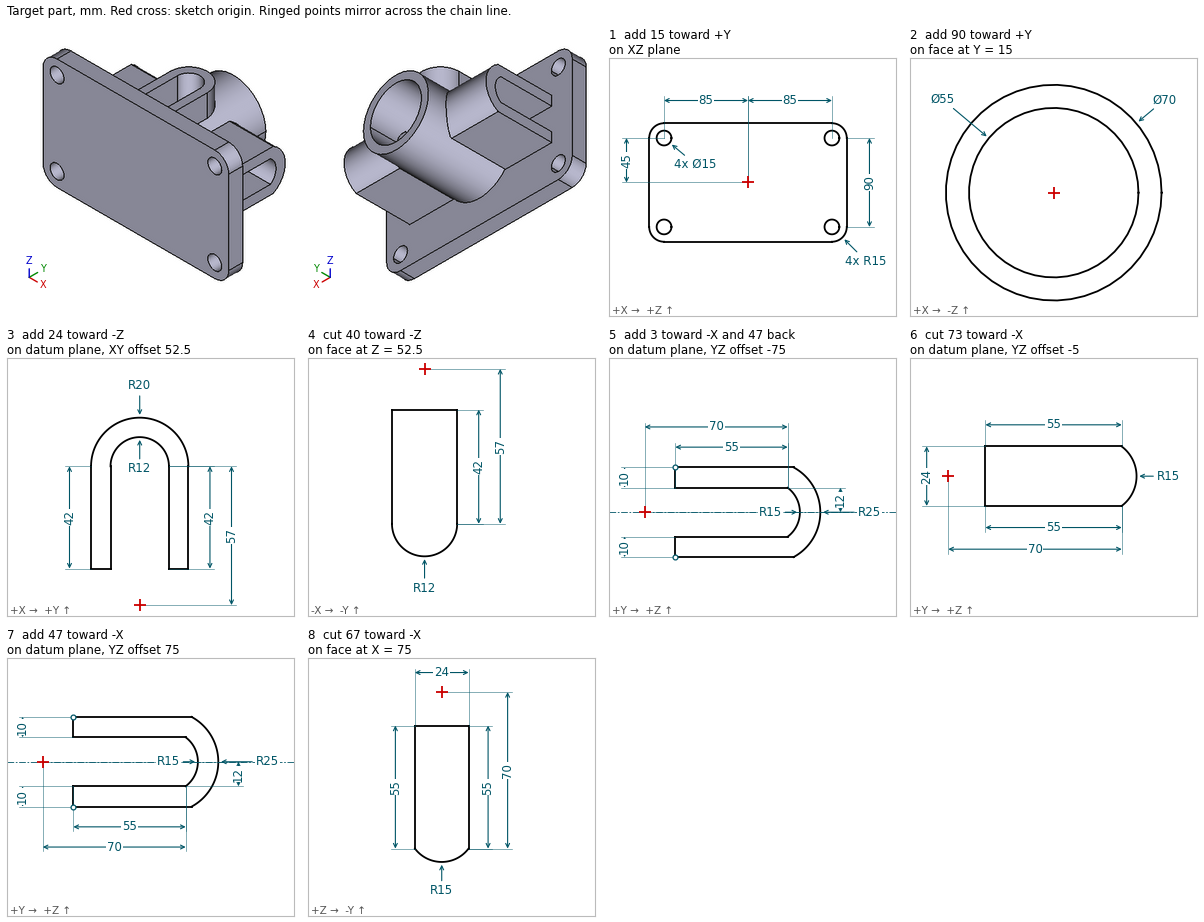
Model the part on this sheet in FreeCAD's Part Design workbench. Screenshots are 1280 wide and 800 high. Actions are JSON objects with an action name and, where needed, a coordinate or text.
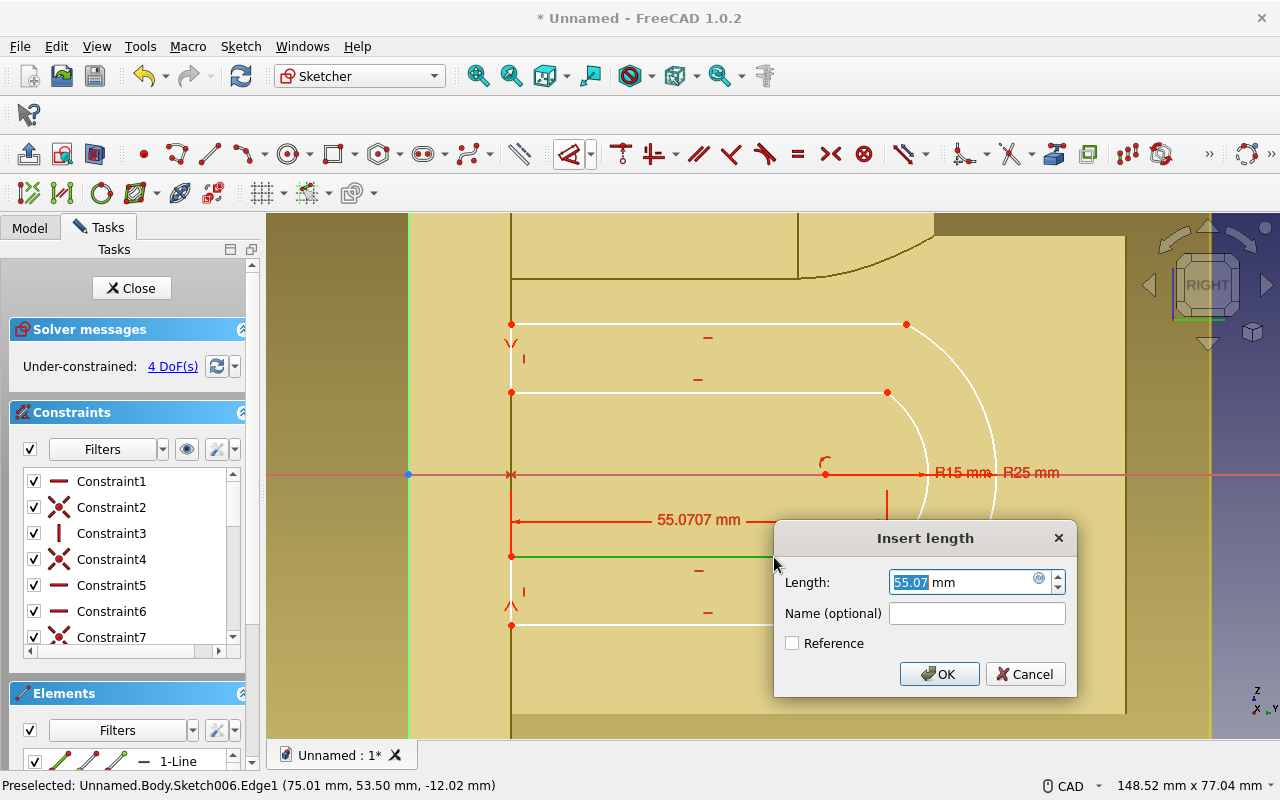
{"action": "type", "text": "55"}
{"action": "key", "text": "Return"}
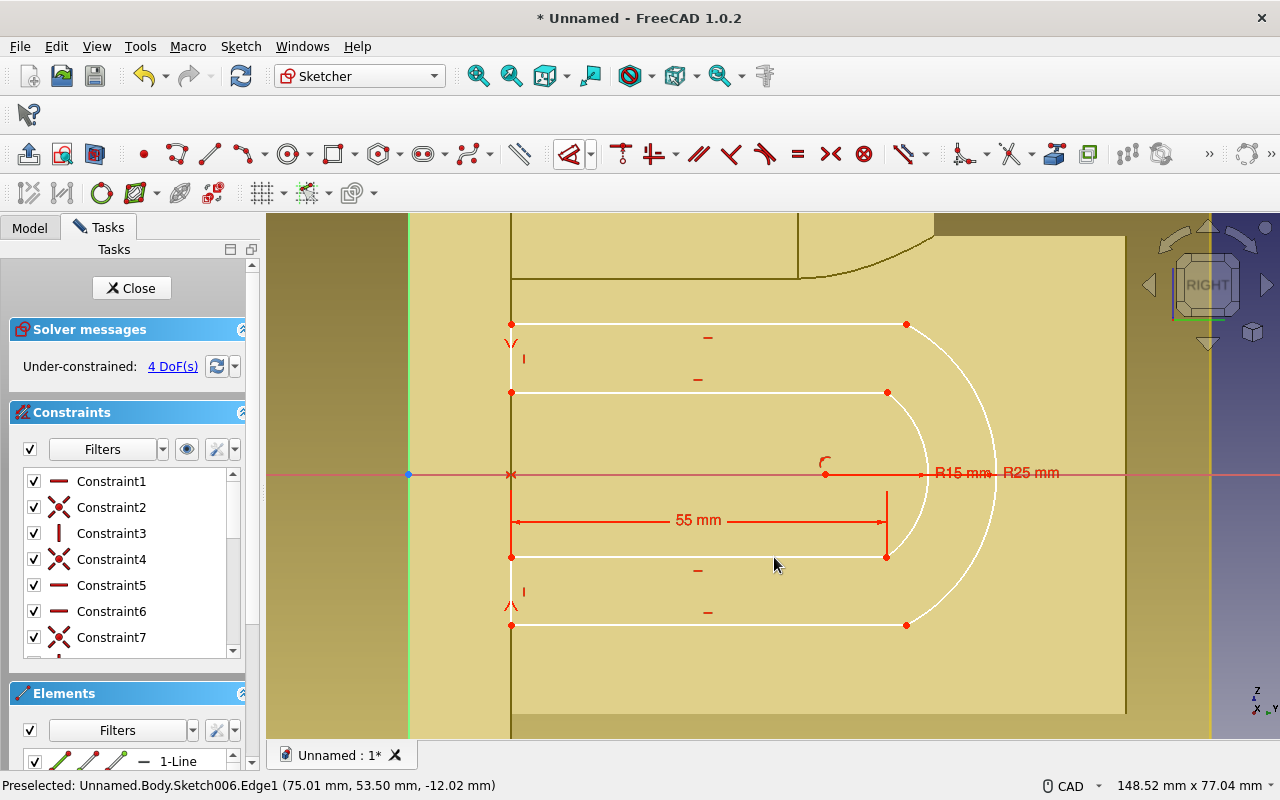
{"action": "left_click", "coordinate": [511, 578]}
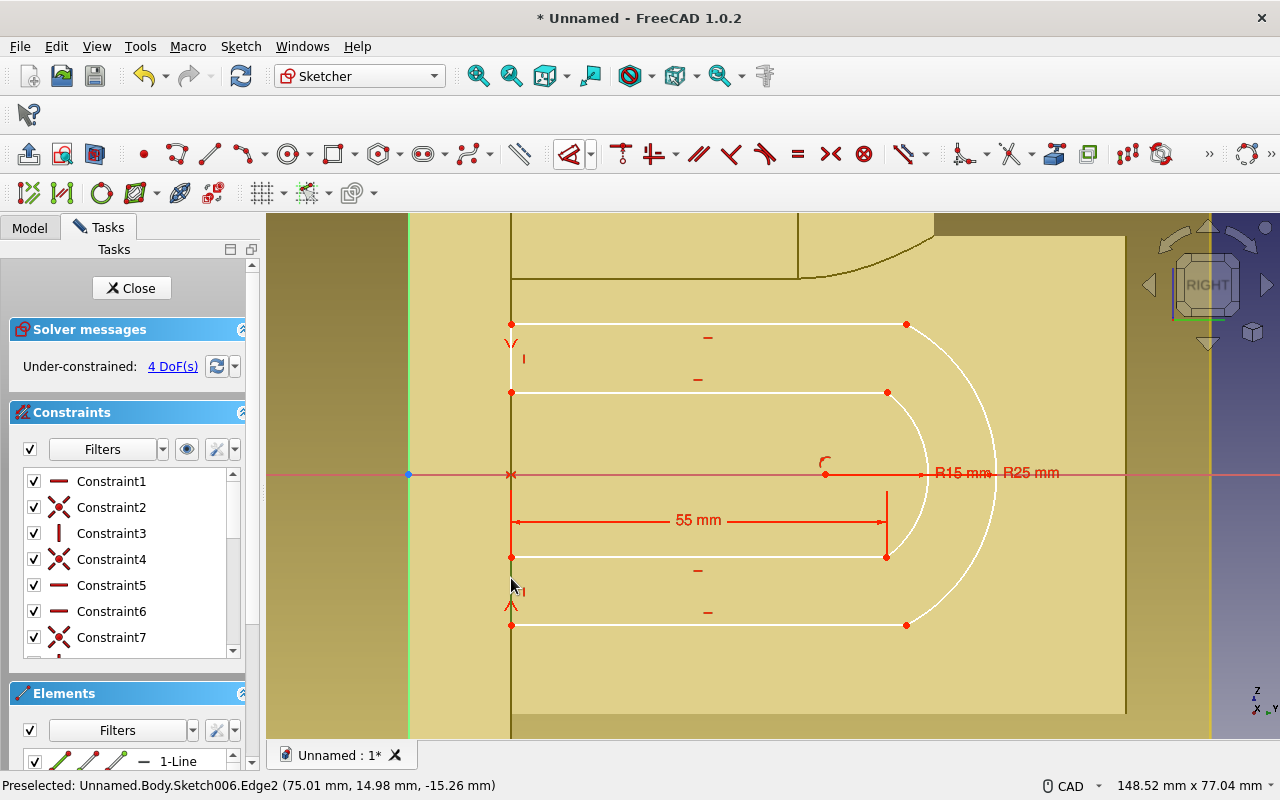
{"action": "key", "text": "i"}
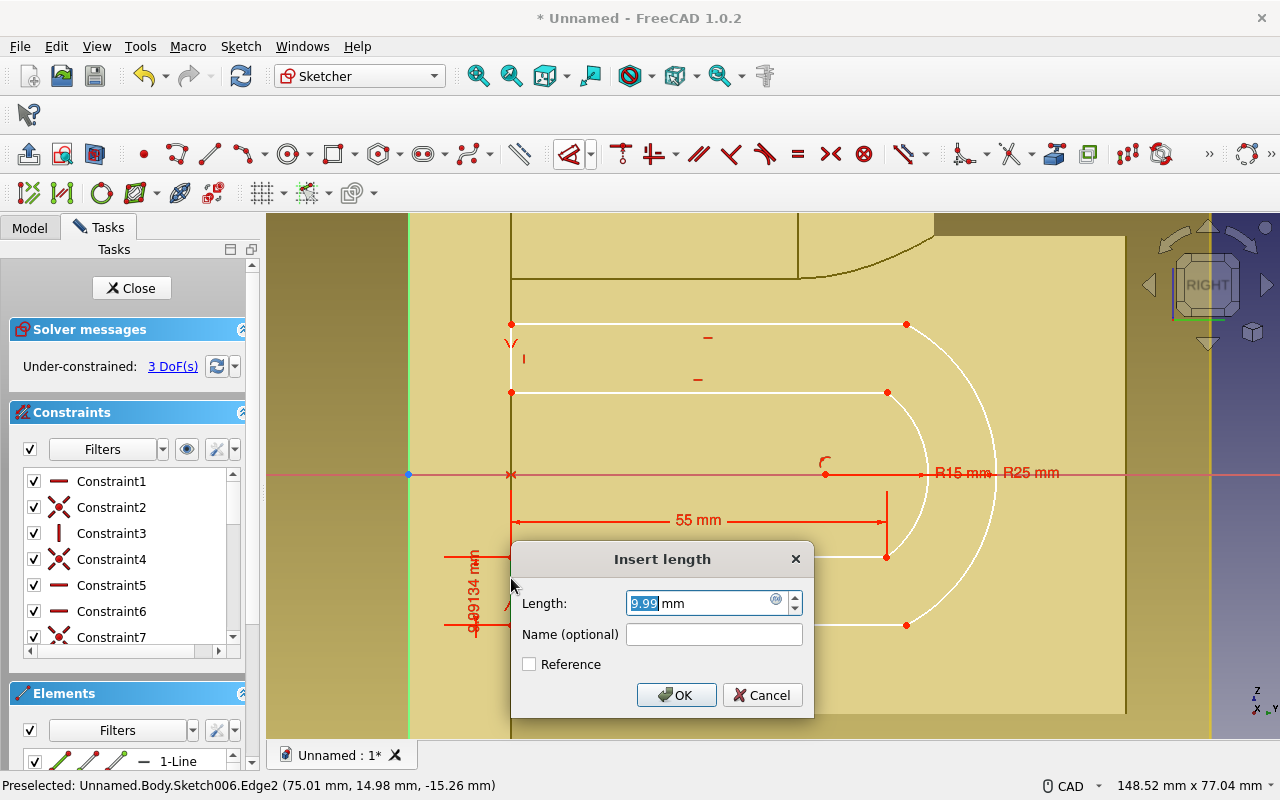
{"action": "type", "text": "10"}
{"action": "key", "text": "Return"}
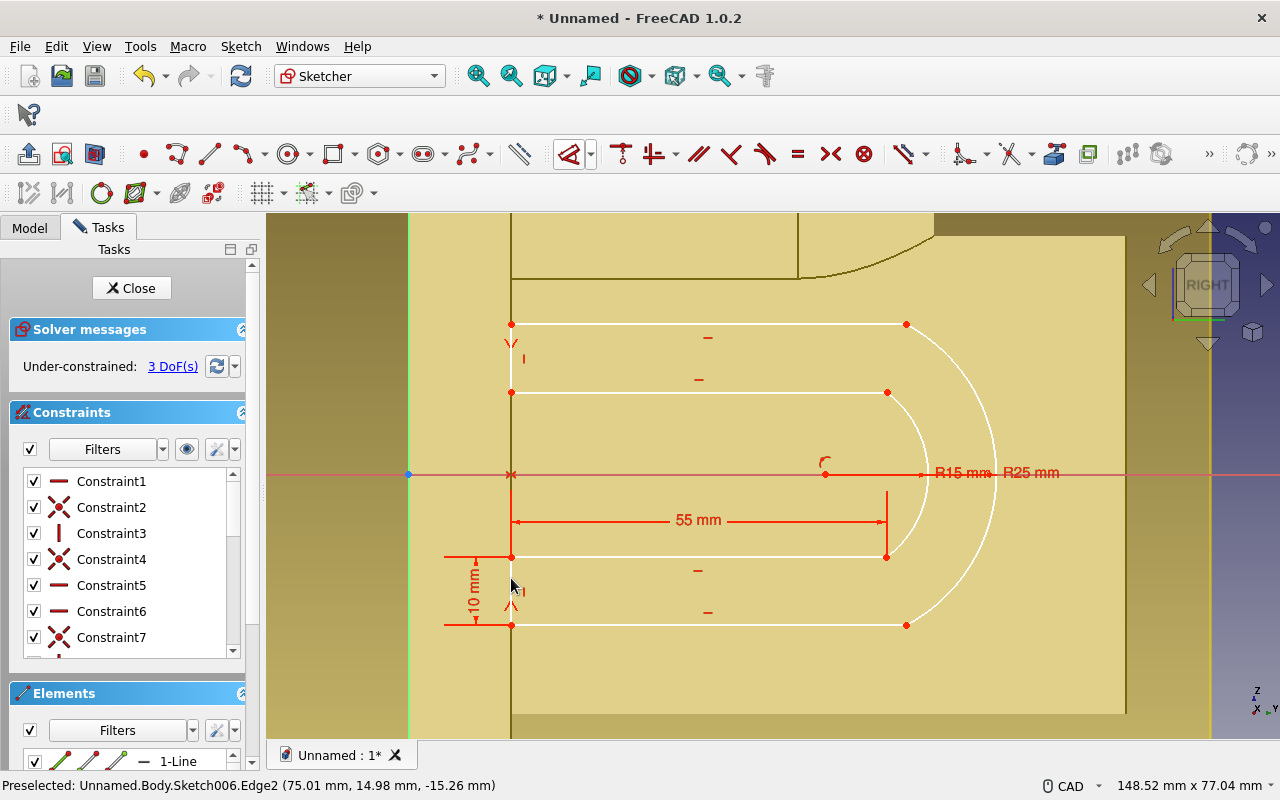
{"action": "left_click", "coordinate": [511, 372]}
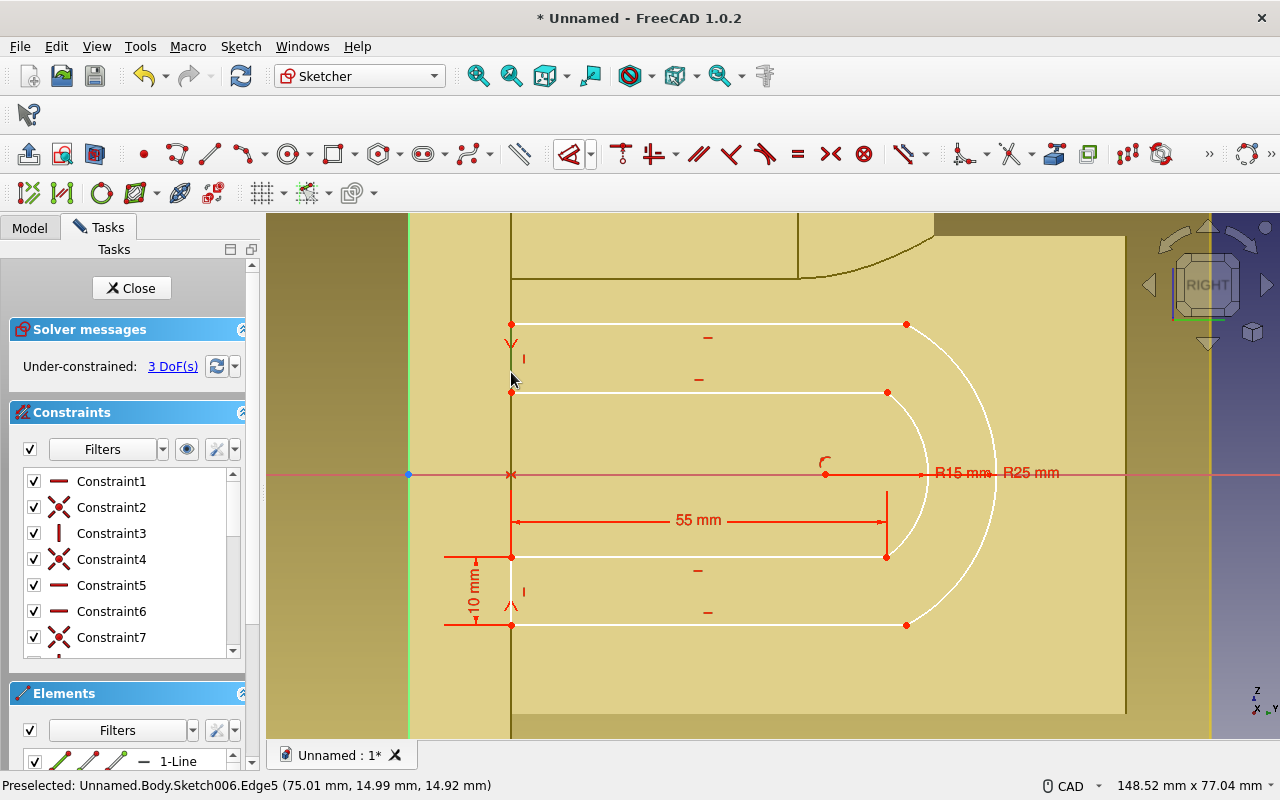
{"action": "left_click", "coordinate": [590, 154]}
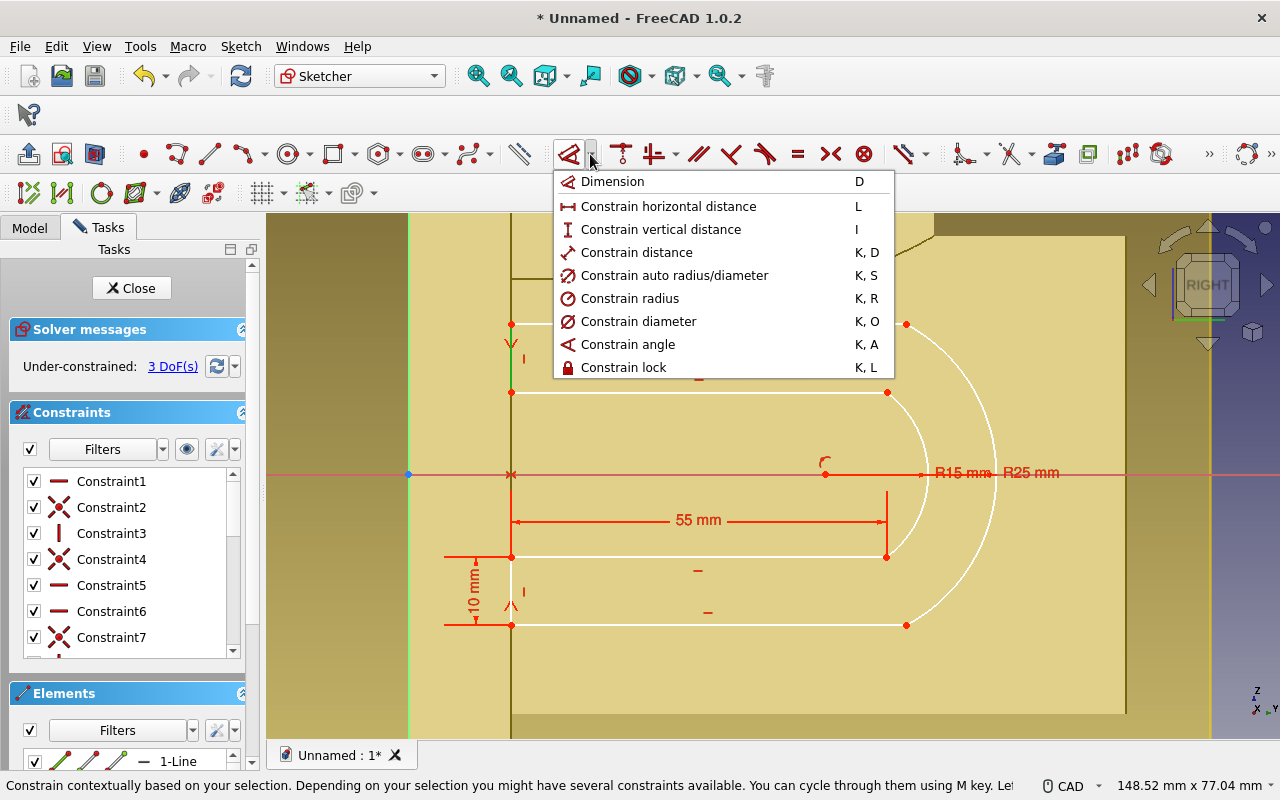
{"action": "left_click", "coordinate": [724, 230]}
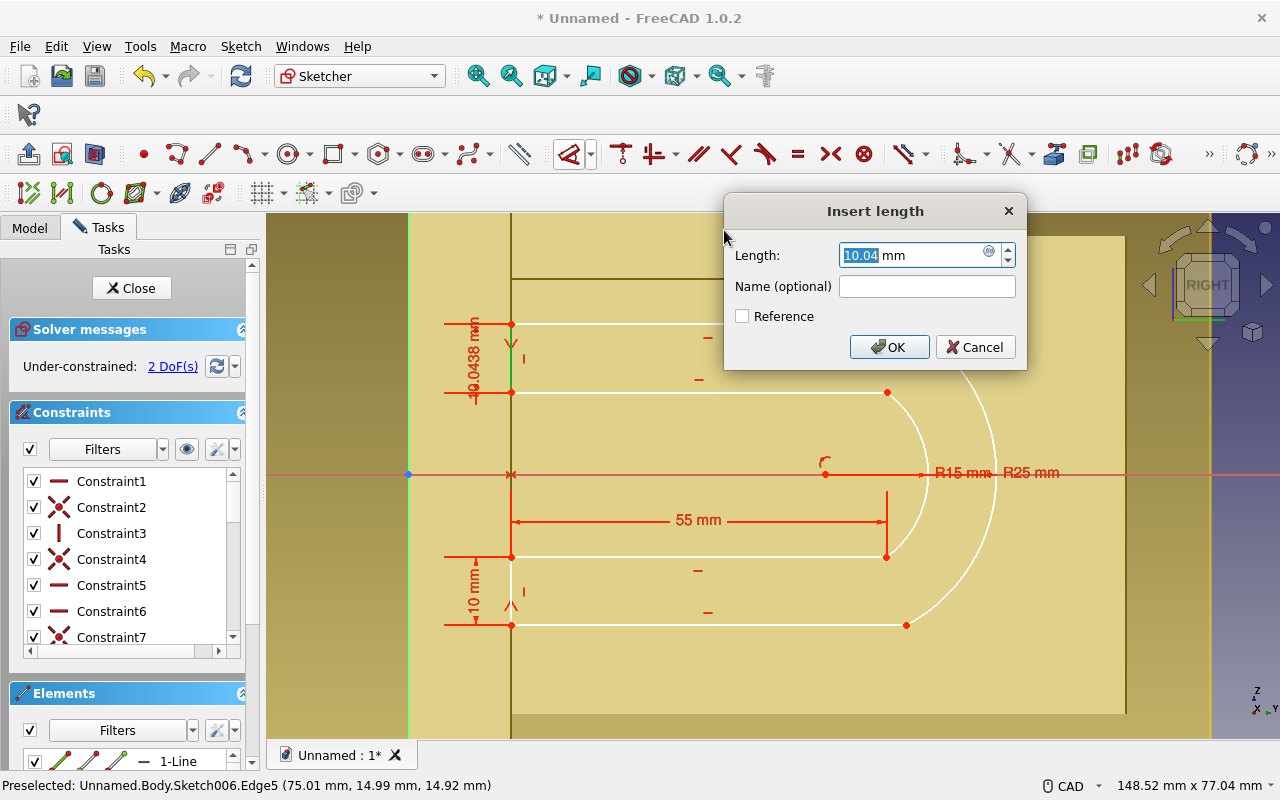
{"action": "type", "text": "10"}
{"action": "key", "text": "Return"}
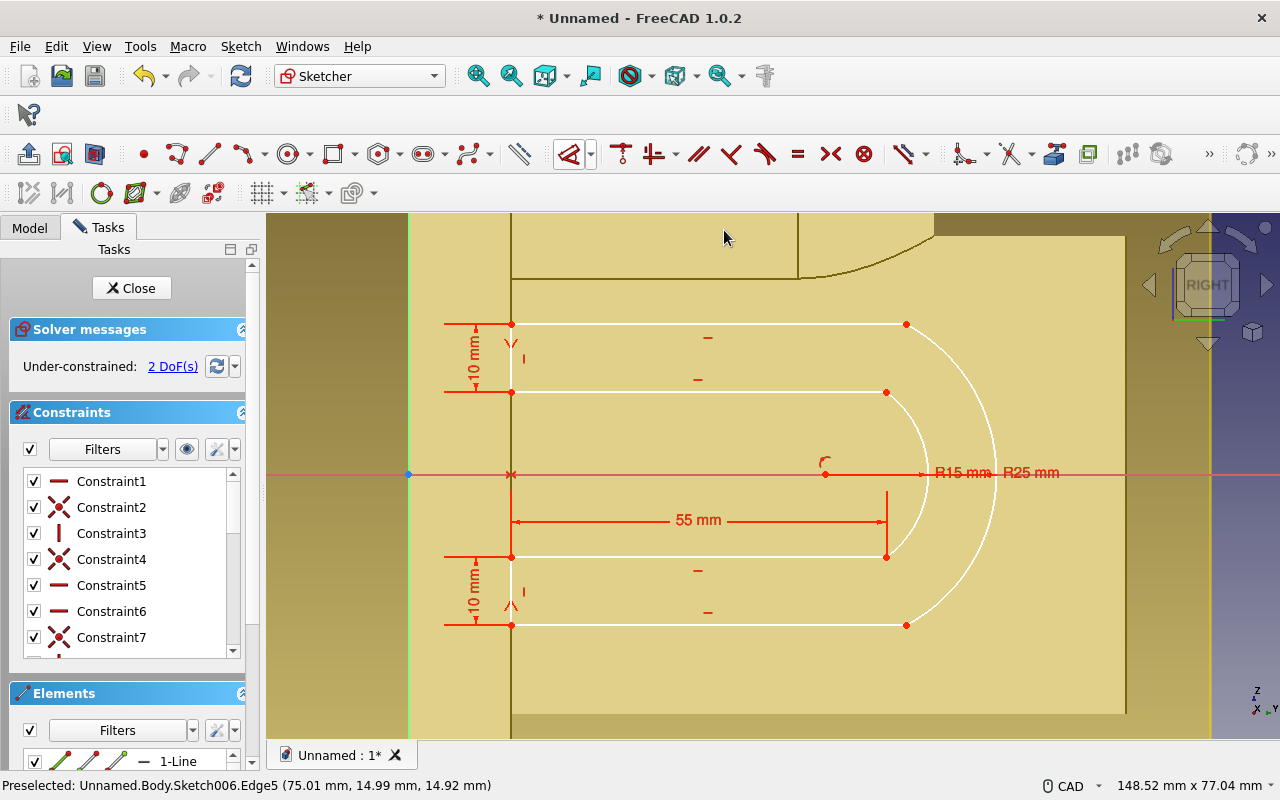
{"action": "left_click", "coordinate": [887, 557]}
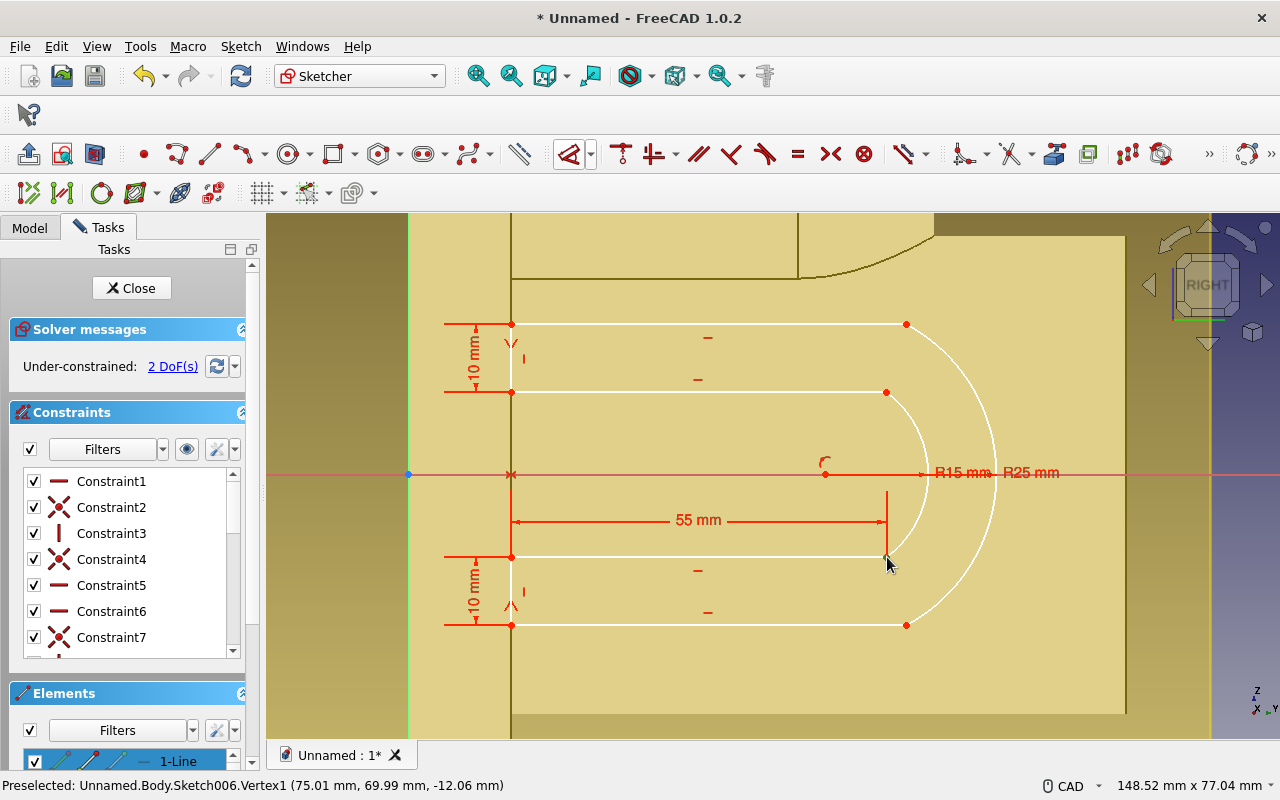
{"action": "key", "text": "l"}